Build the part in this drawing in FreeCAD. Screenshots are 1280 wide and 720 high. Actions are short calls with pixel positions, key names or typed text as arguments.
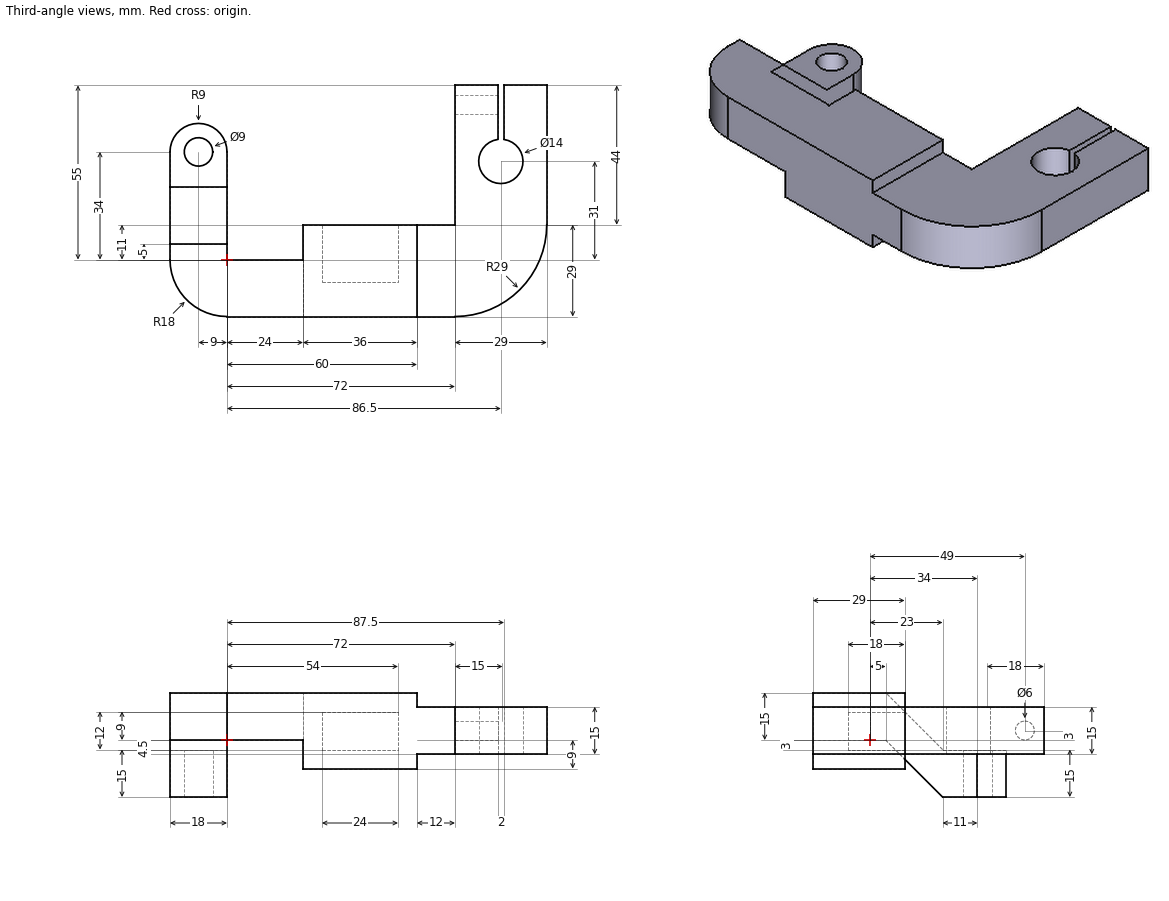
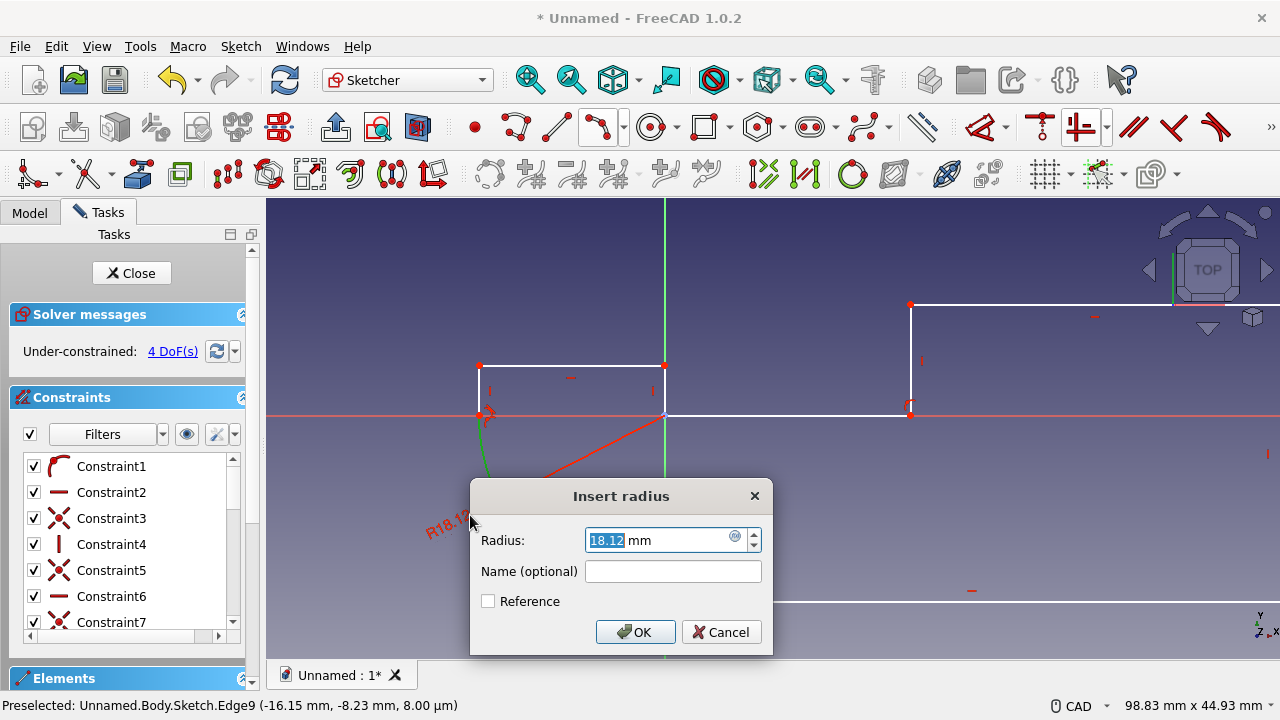
text(18)
key(Return)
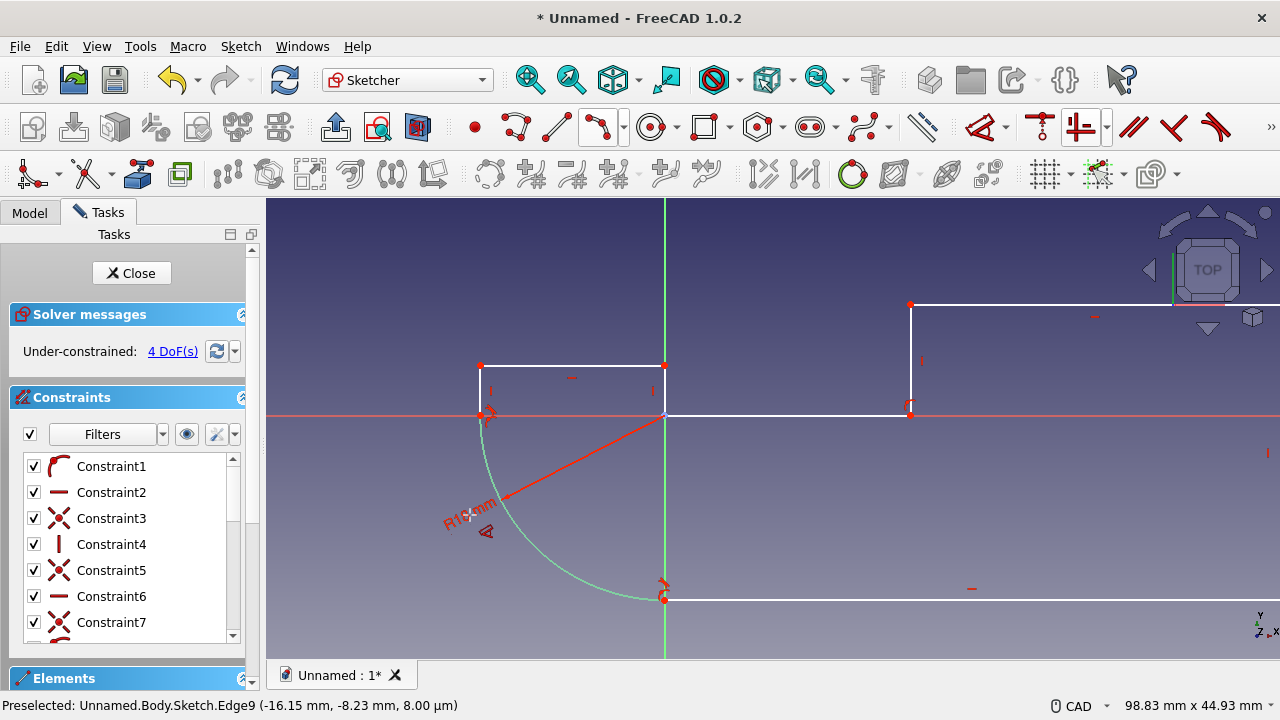
click(665, 401)
click(631, 391)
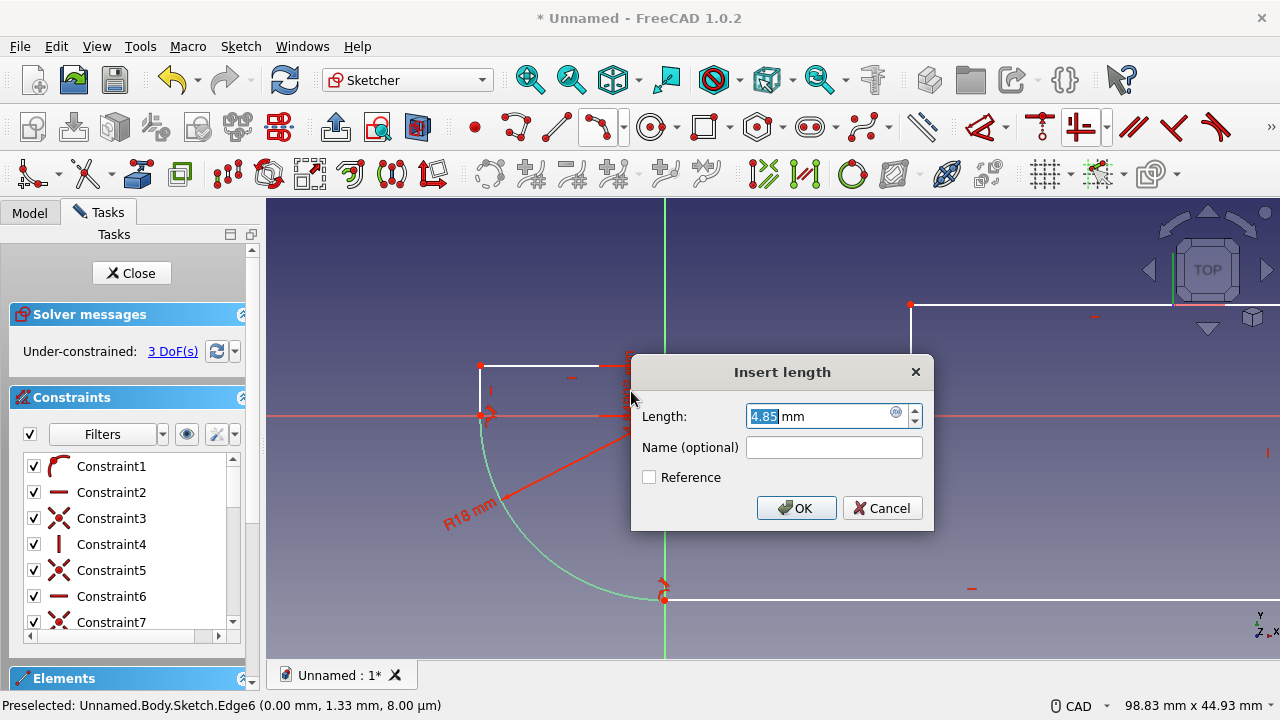
text(5)
key(Return)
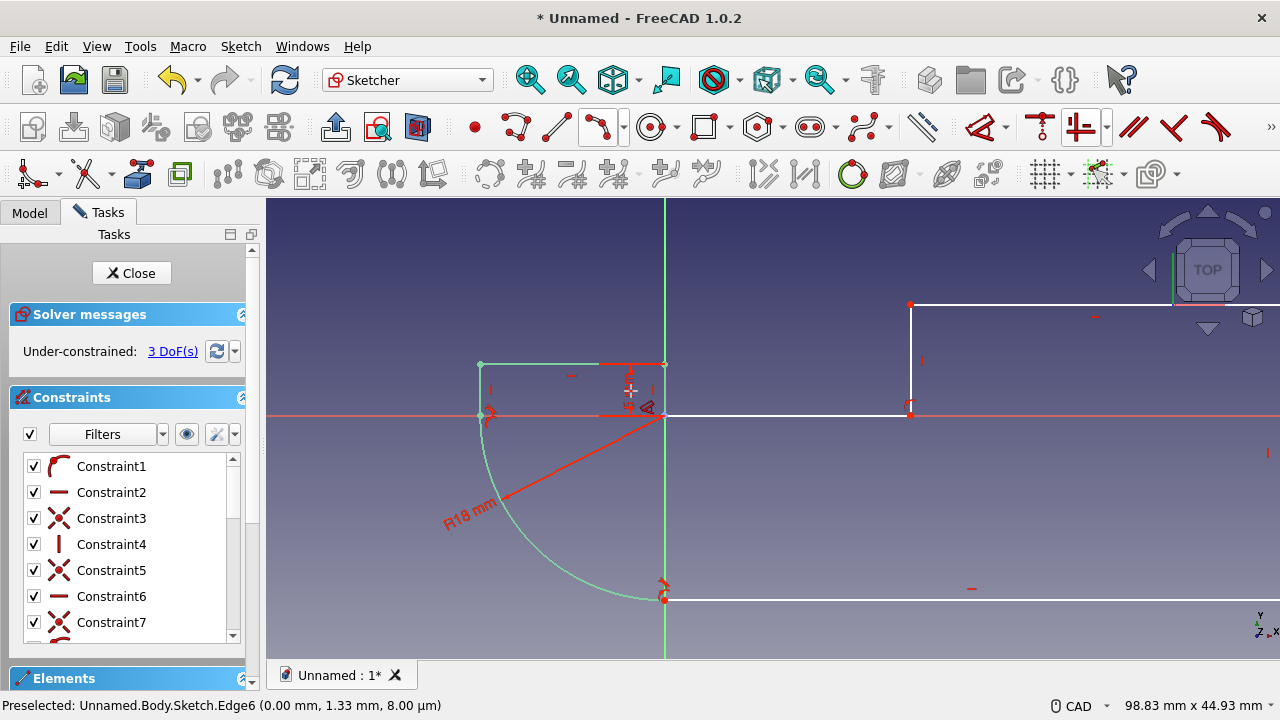
click(850, 600)
click(890, 566)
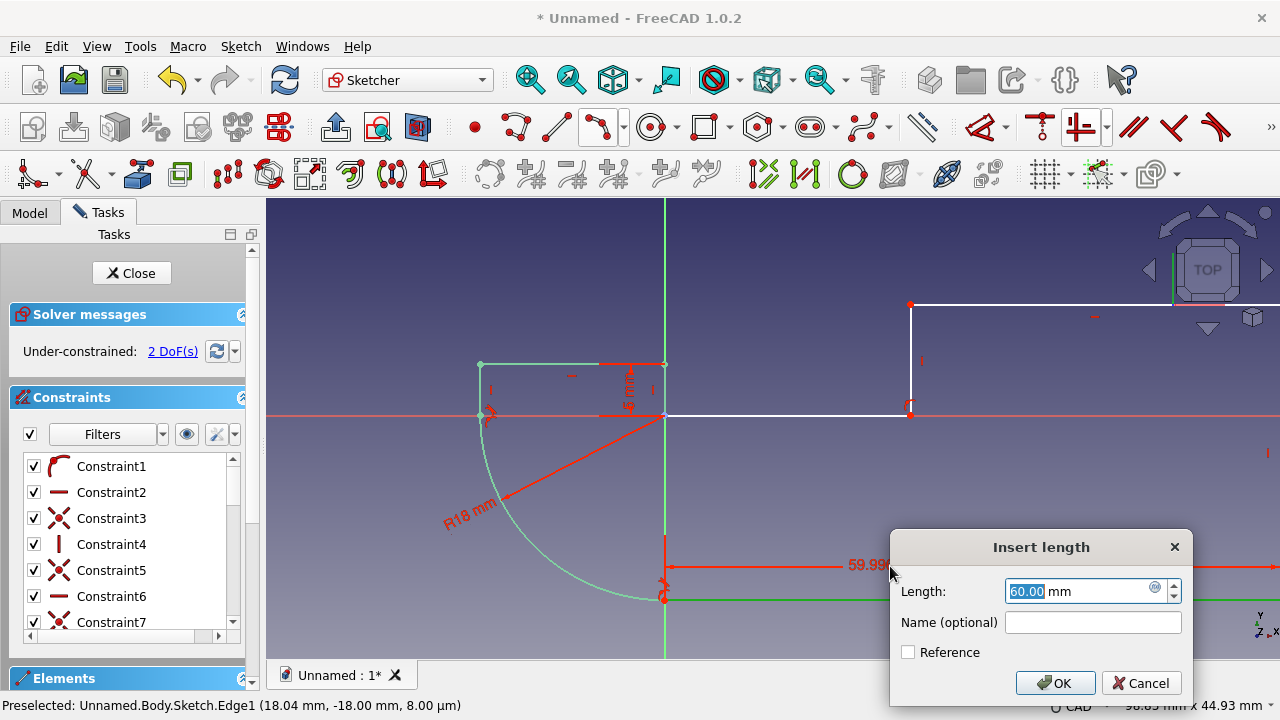
text(60)
key(Return)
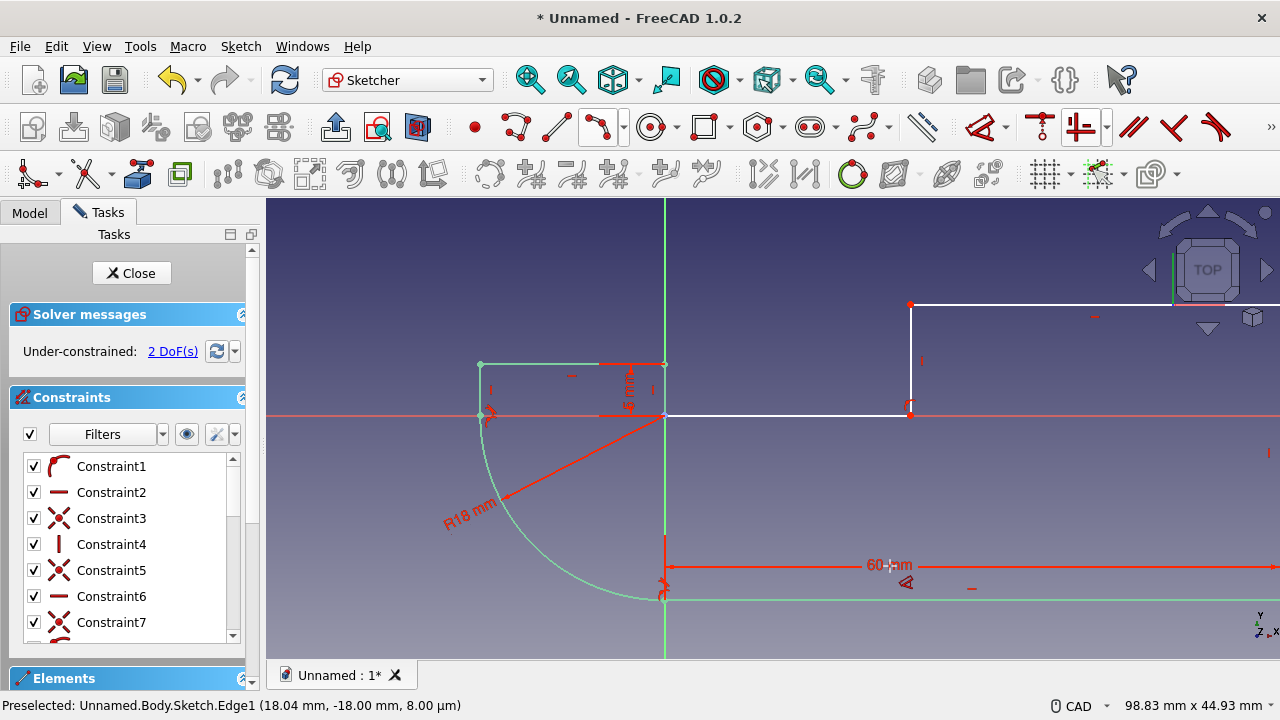
scroll(347, 382, down, 2)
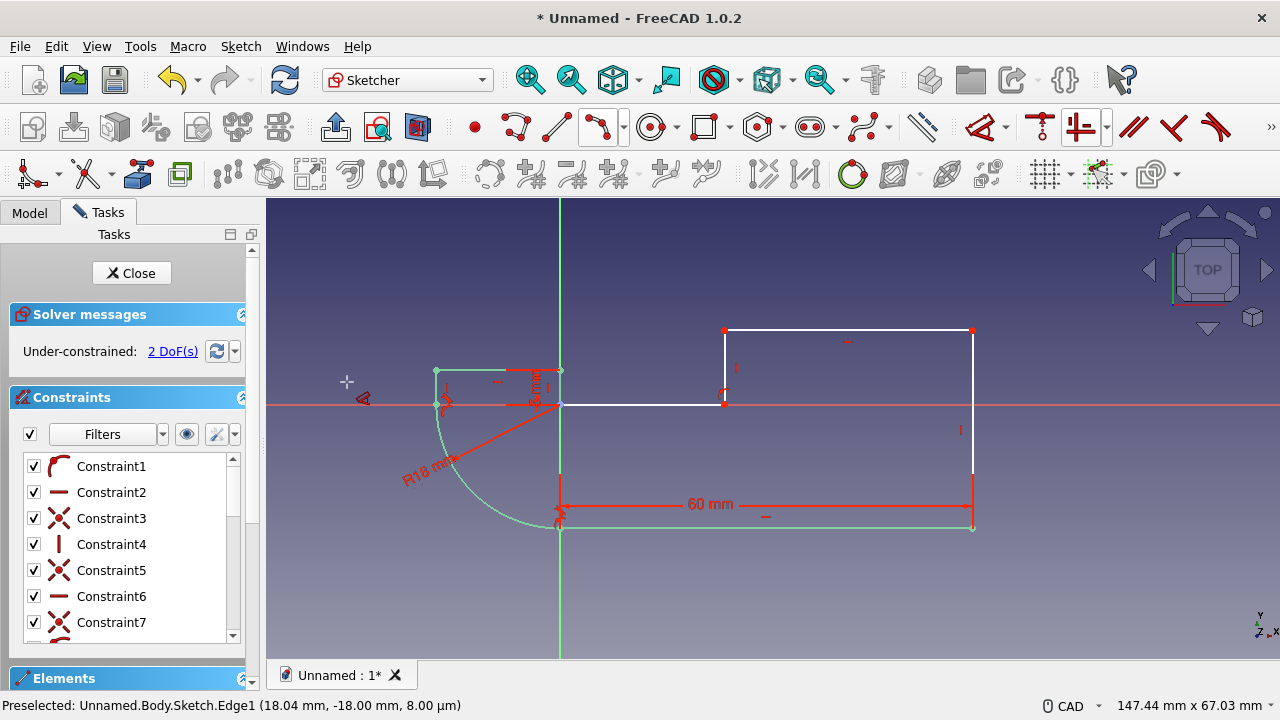
click(973, 469)
click(1007, 429)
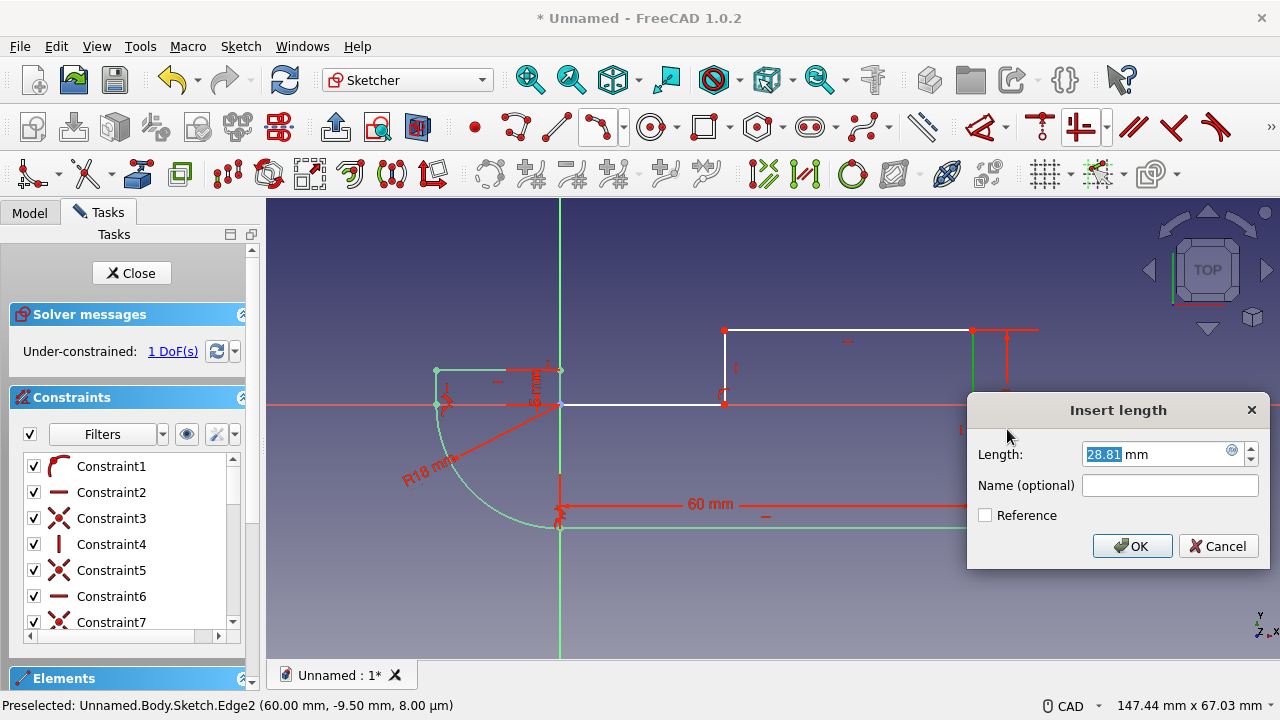
text(29)
key(Return)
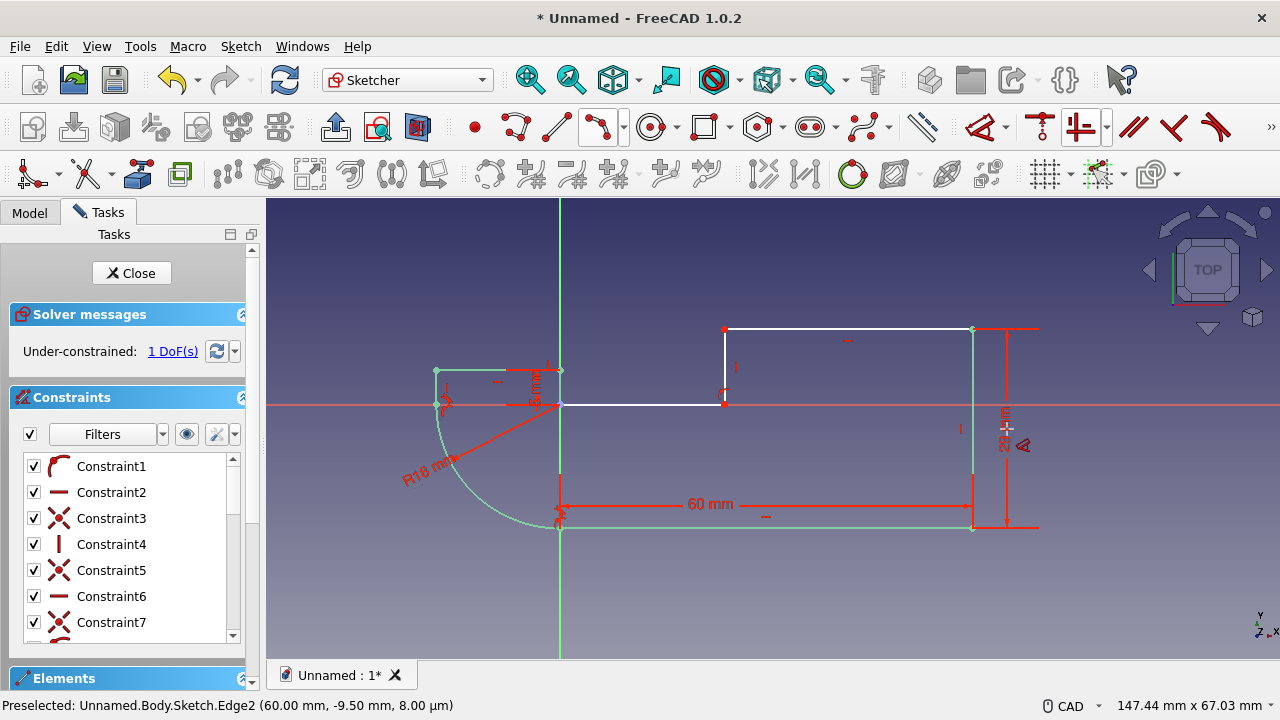
click(898, 329)
click(849, 295)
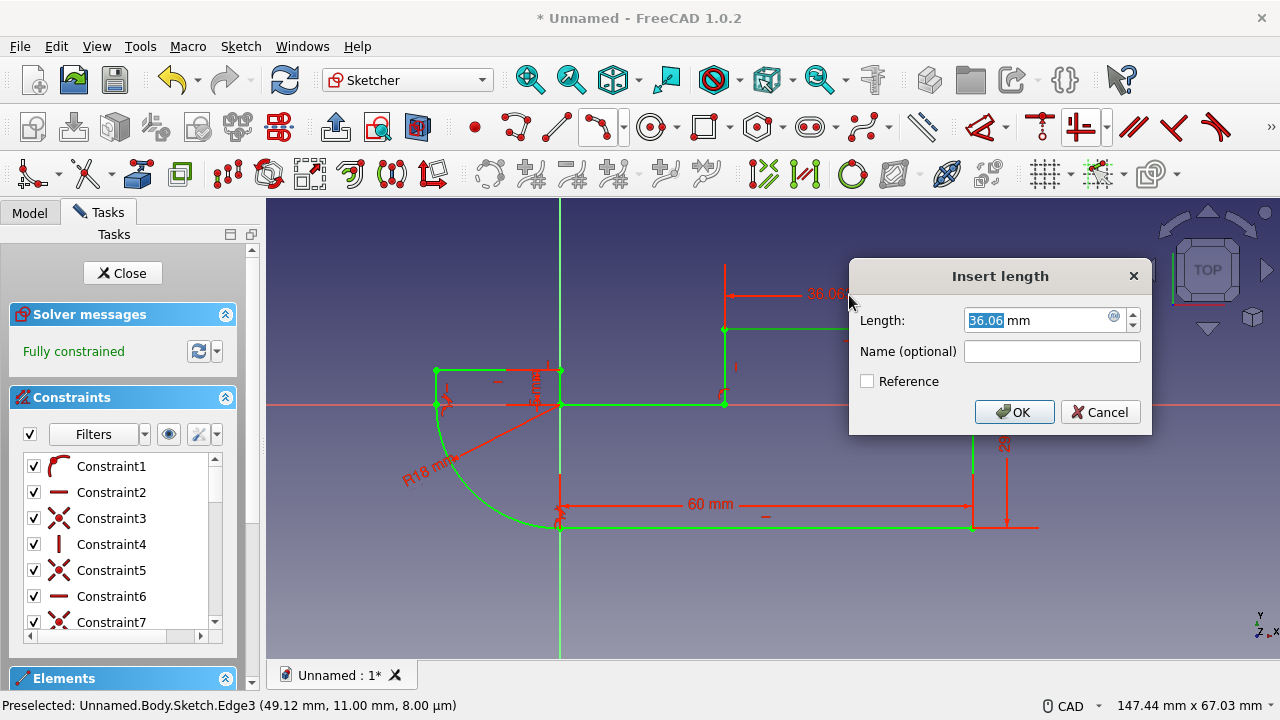
text(36)
key(Return)
key(Escape)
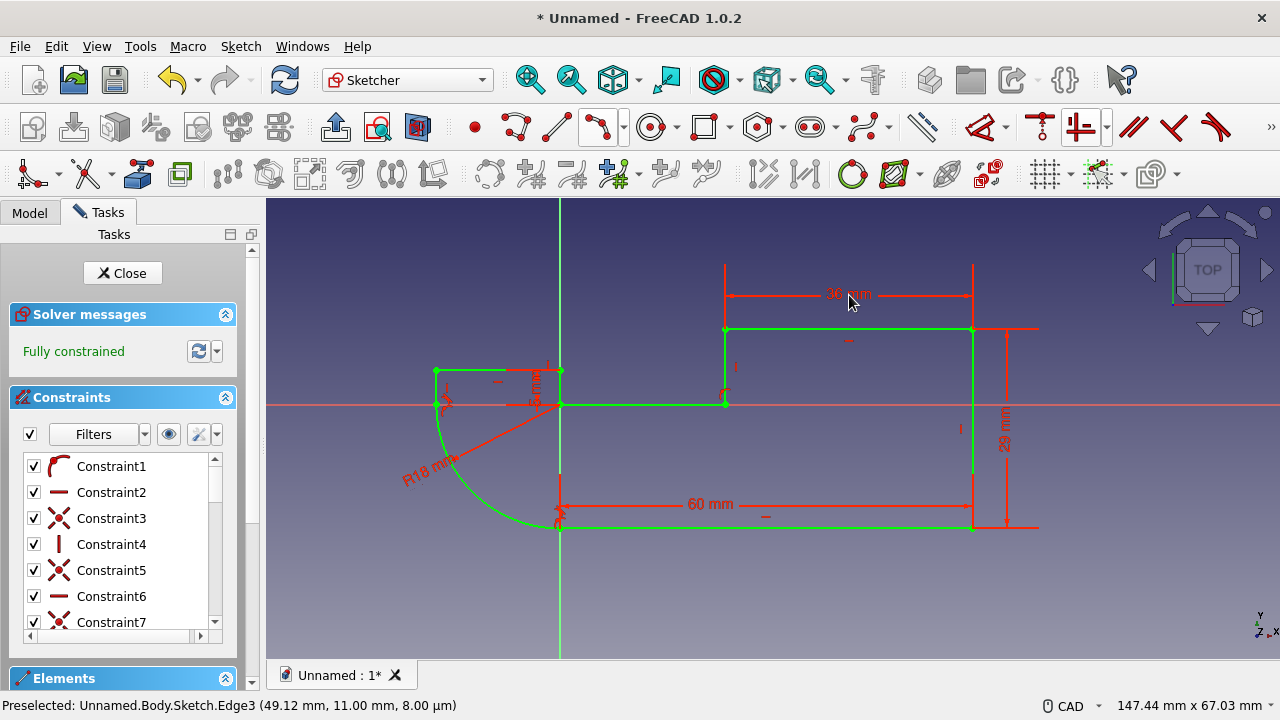
click(123, 273)